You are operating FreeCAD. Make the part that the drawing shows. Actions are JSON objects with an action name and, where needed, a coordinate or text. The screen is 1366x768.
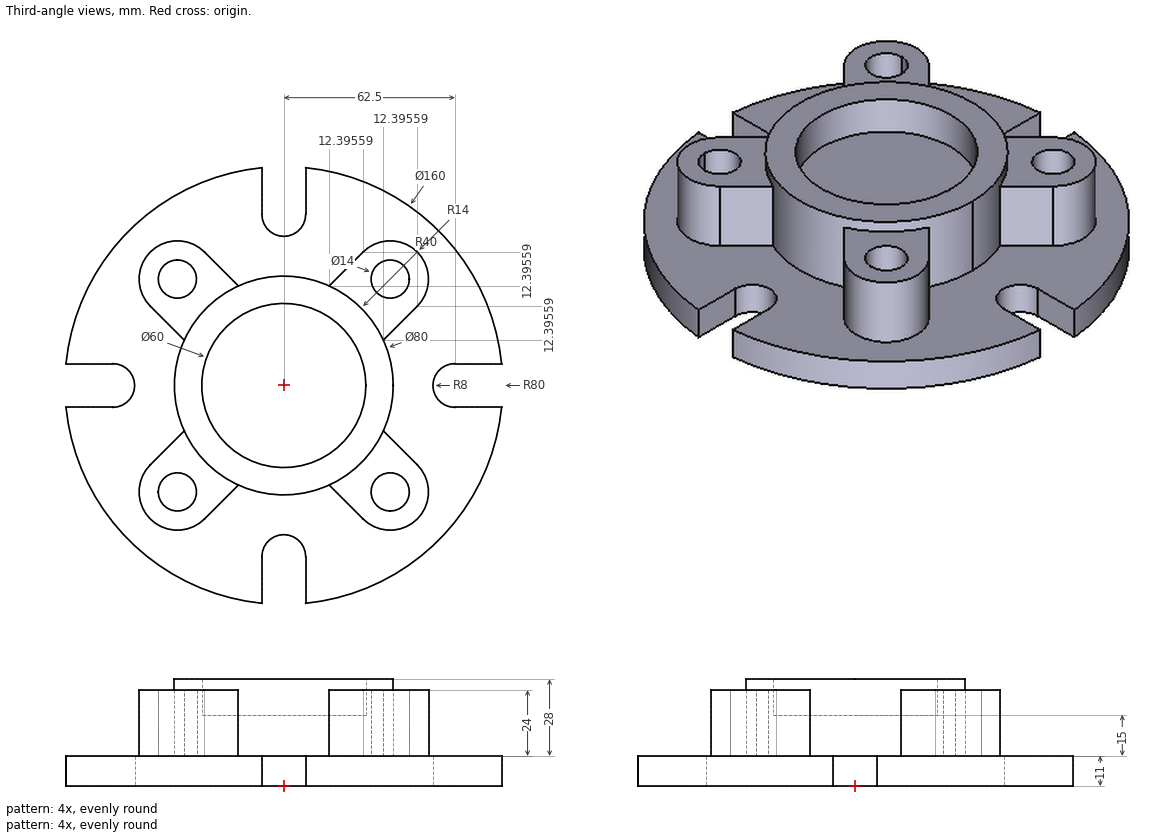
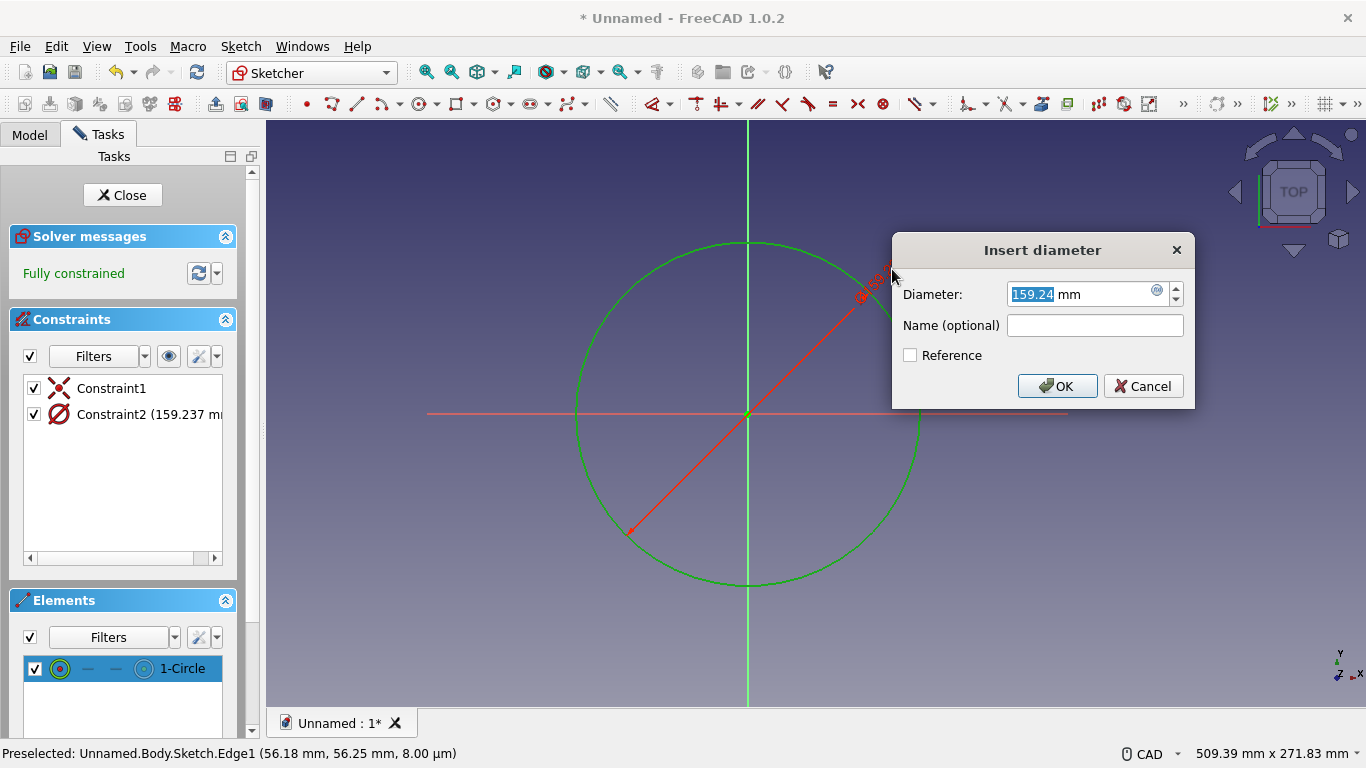
{"action": "type", "text": "160"}
{"action": "key", "text": "Return"}
{"action": "key", "text": "Escape"}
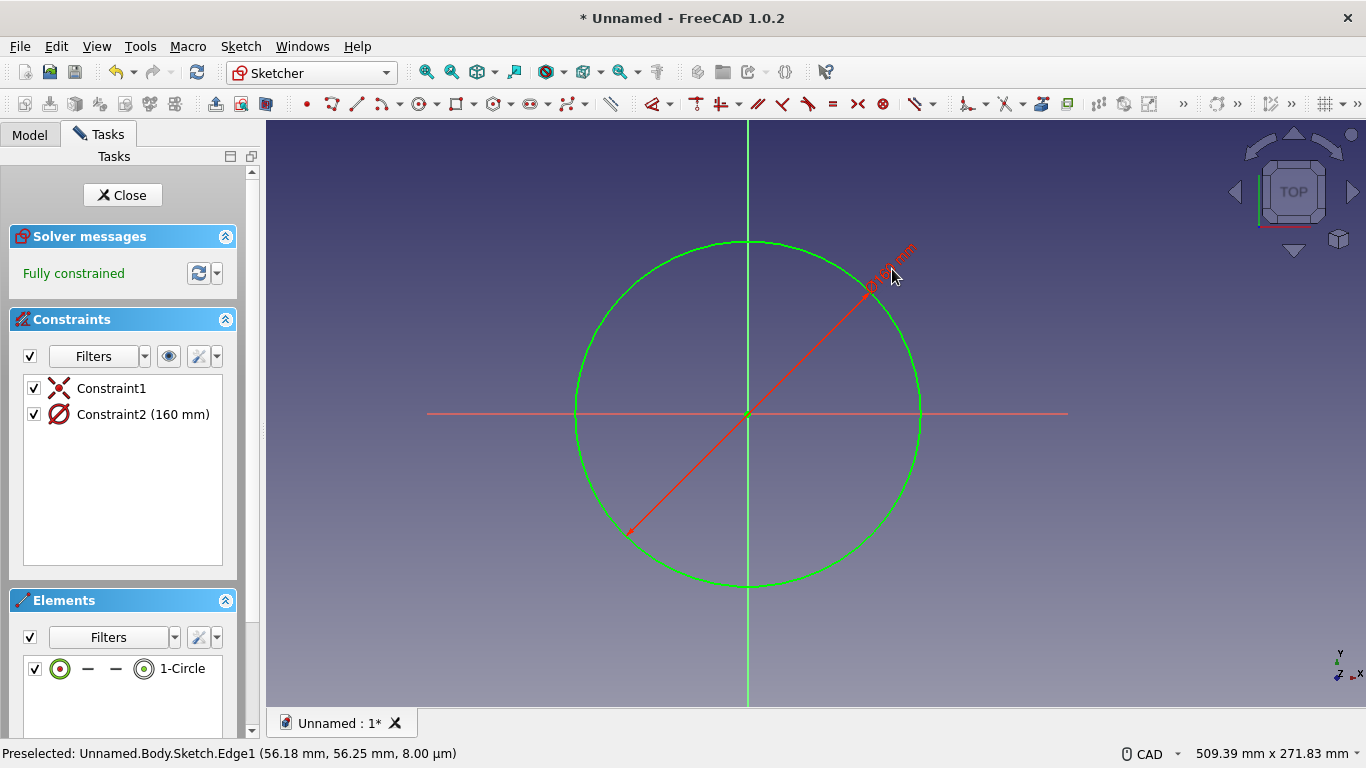
{"action": "left_click", "coordinate": [123, 195]}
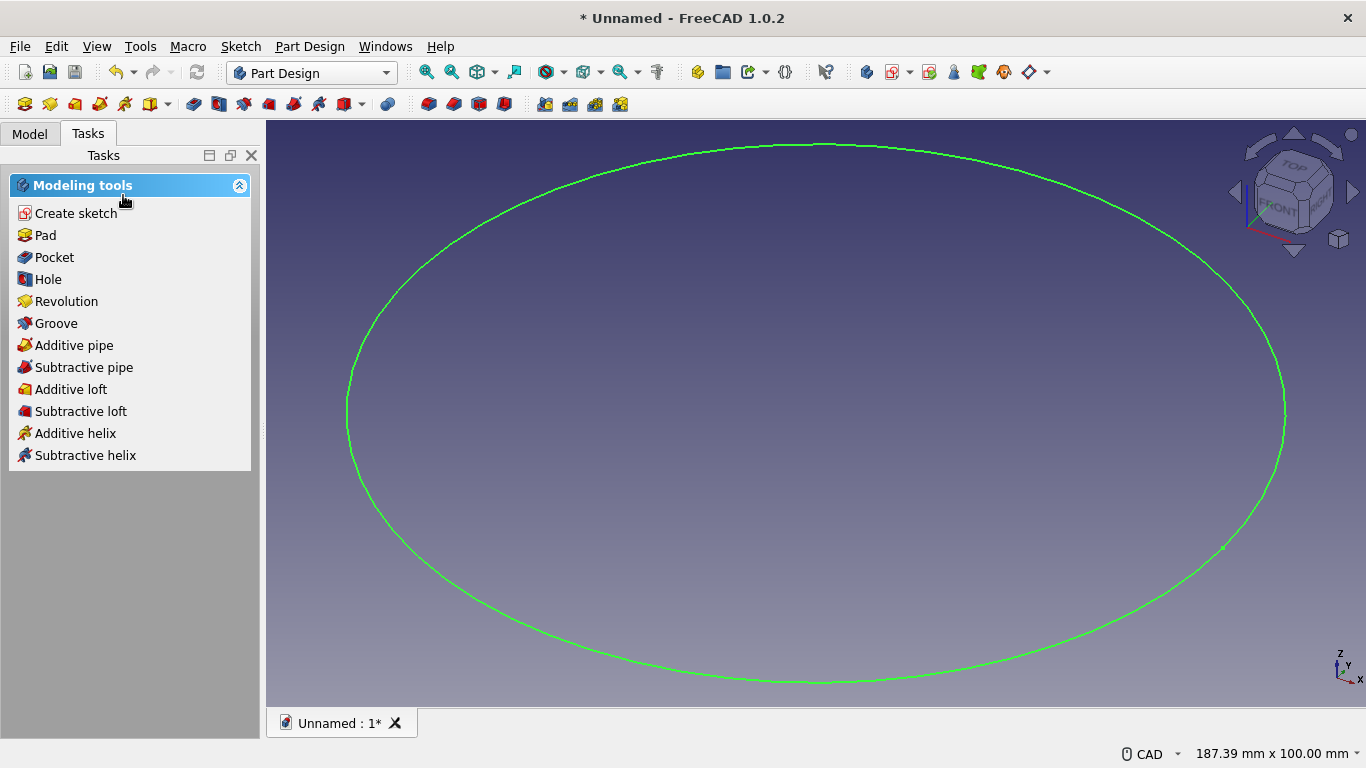
{"action": "left_click", "coordinate": [25, 104]}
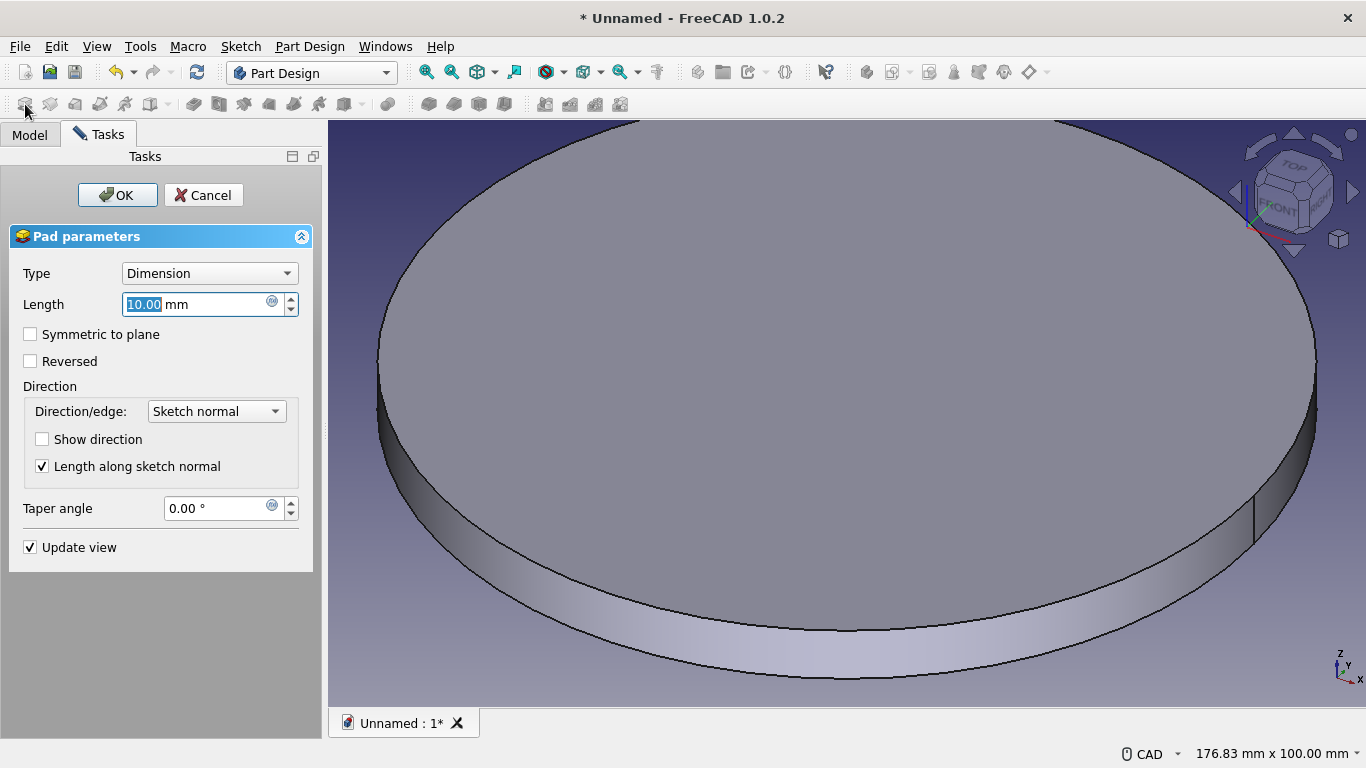
{"action": "type", "text": "11"}
{"action": "key", "text": "Tab"}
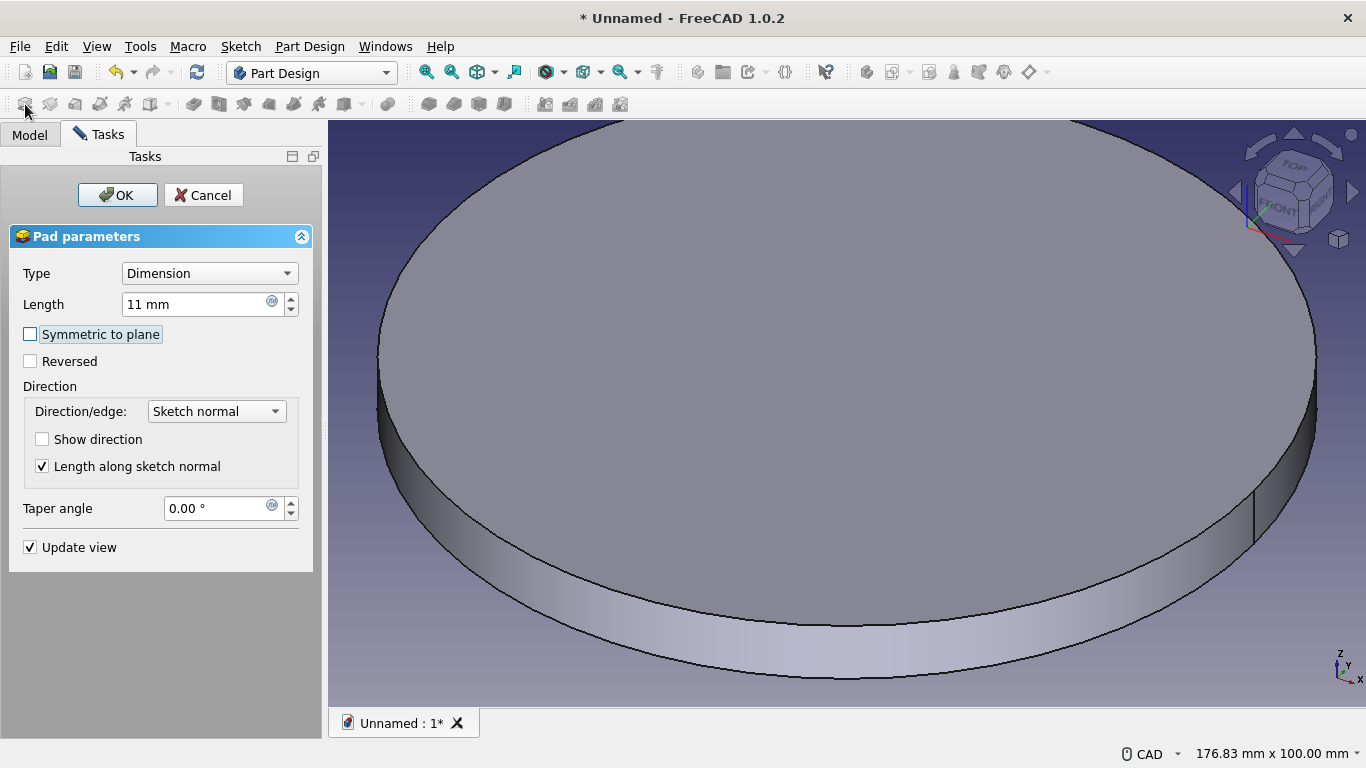
{"action": "left_click", "coordinate": [118, 195]}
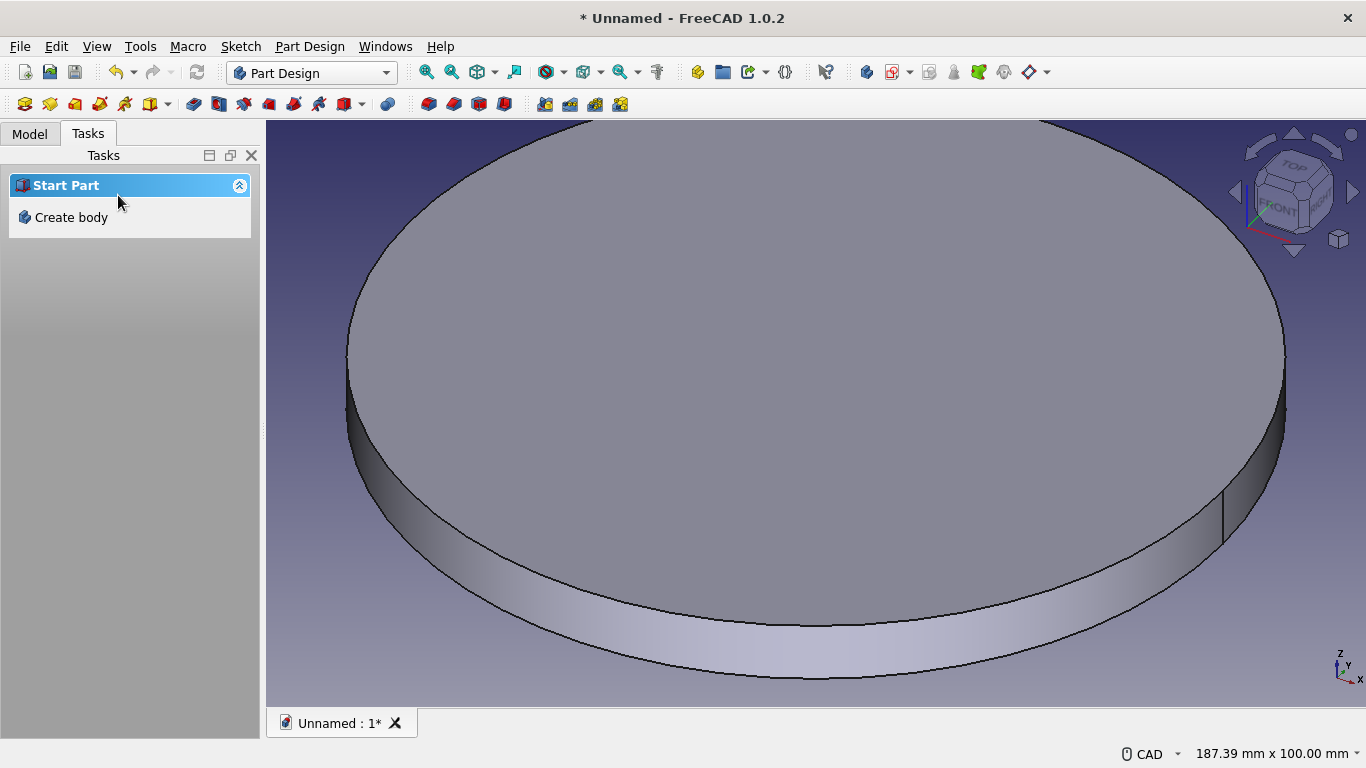
{"action": "key", "text": "v f"}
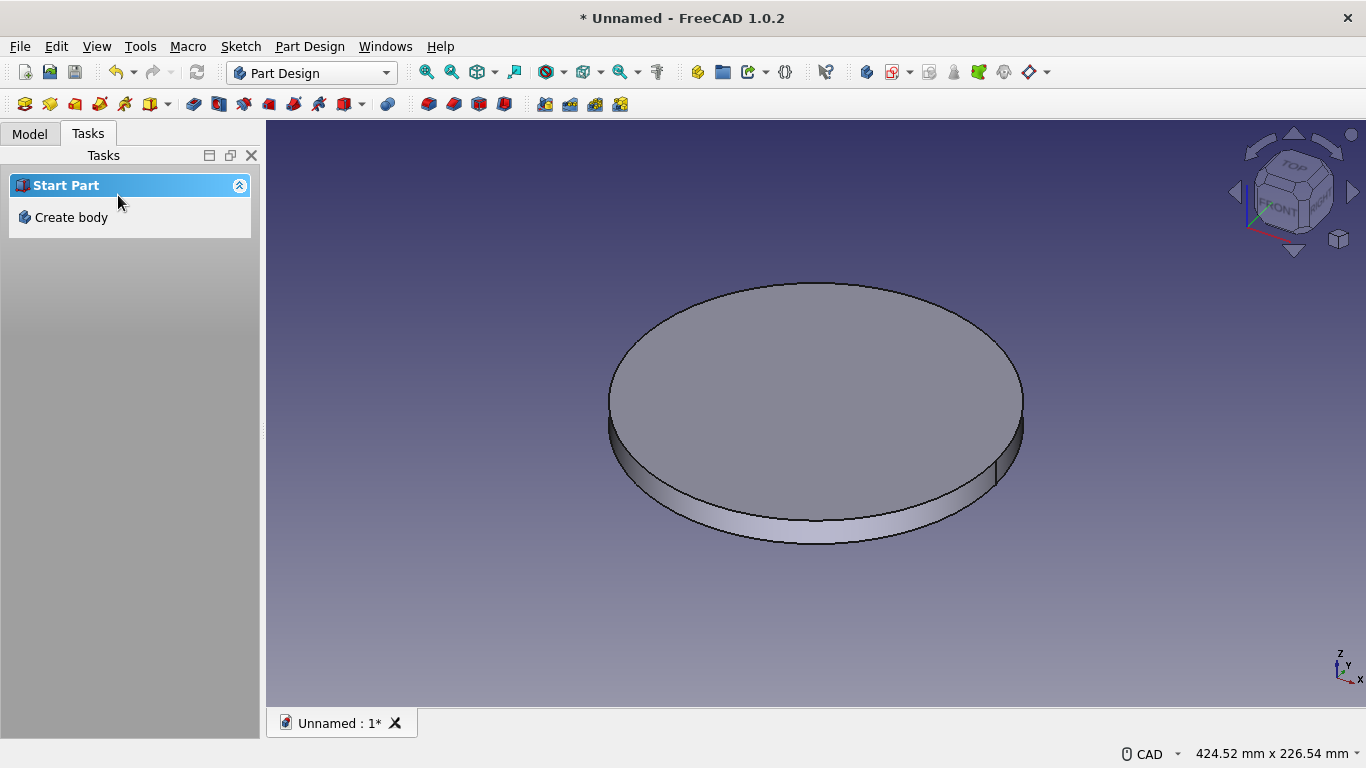
{"action": "left_click", "coordinate": [816, 401]}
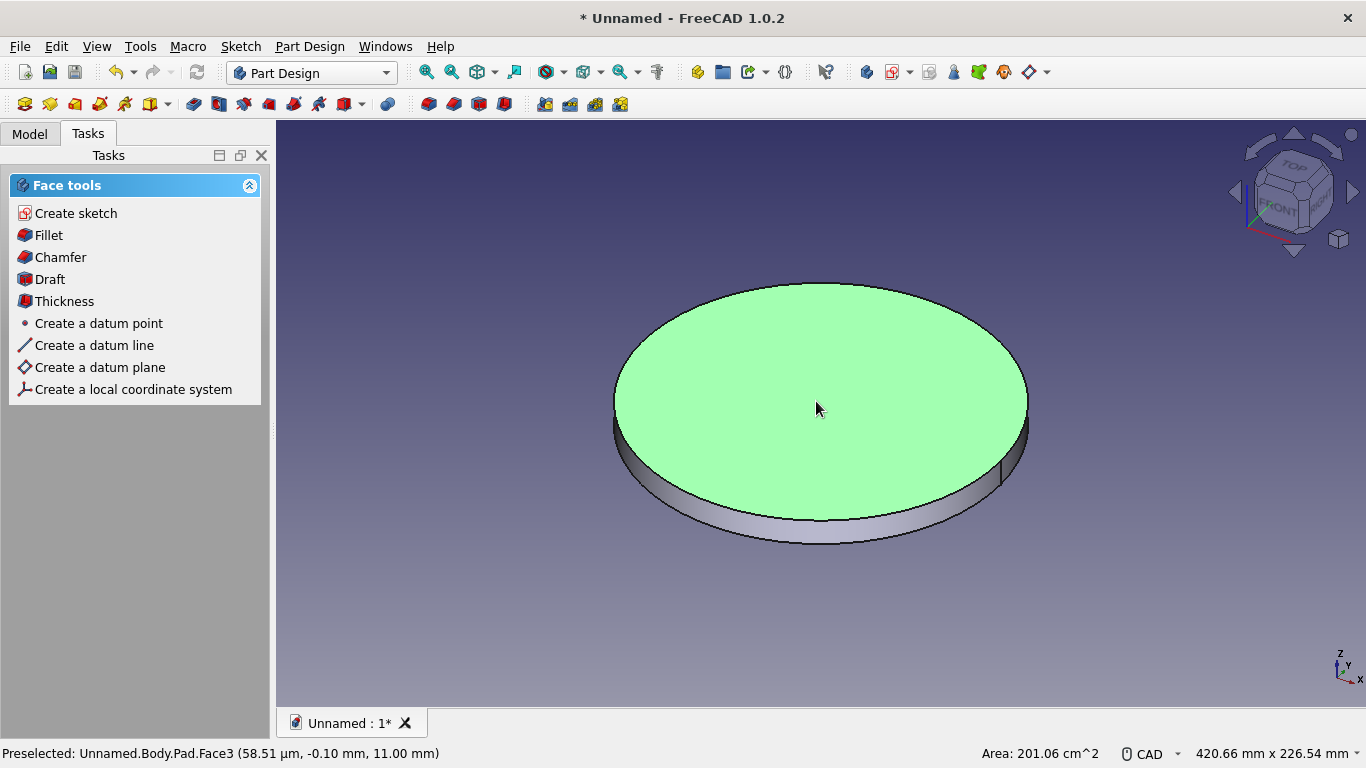
{"action": "left_click", "coordinate": [892, 72]}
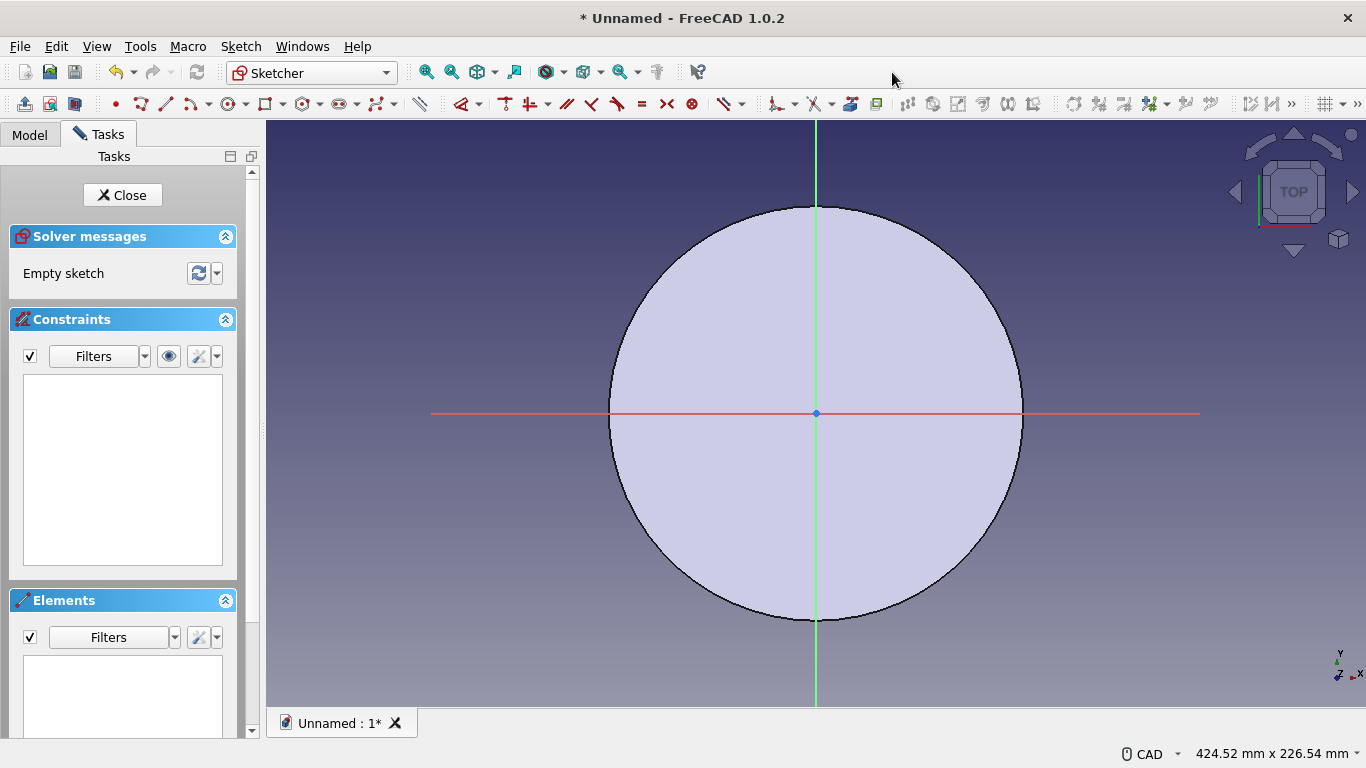
{"action": "scroll", "coordinate": [899, 414], "scroll_direction": "up", "scroll_amount": 3}